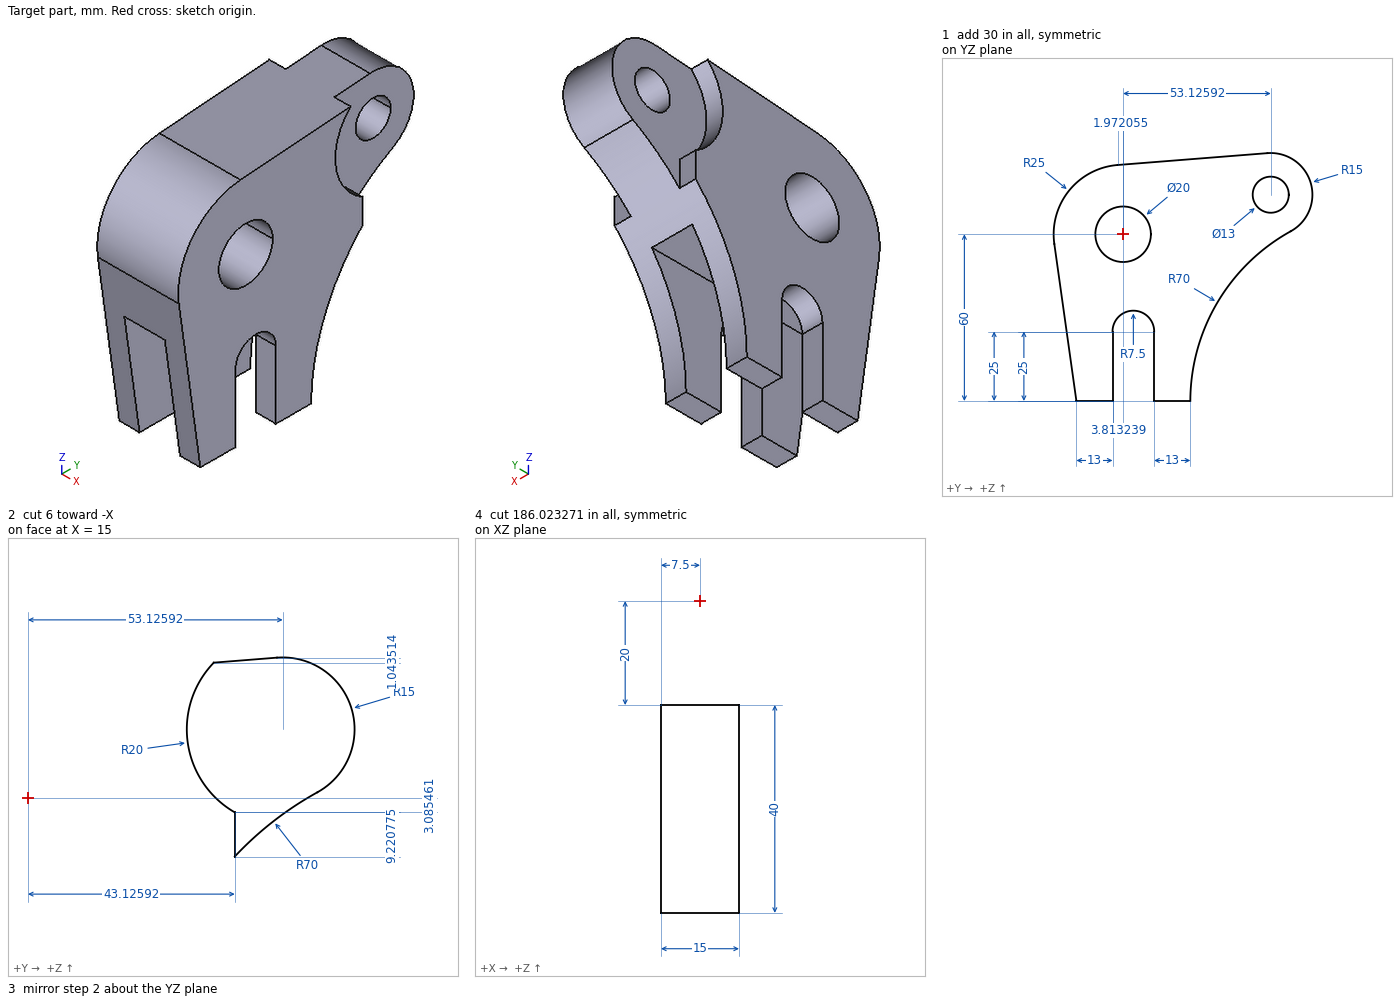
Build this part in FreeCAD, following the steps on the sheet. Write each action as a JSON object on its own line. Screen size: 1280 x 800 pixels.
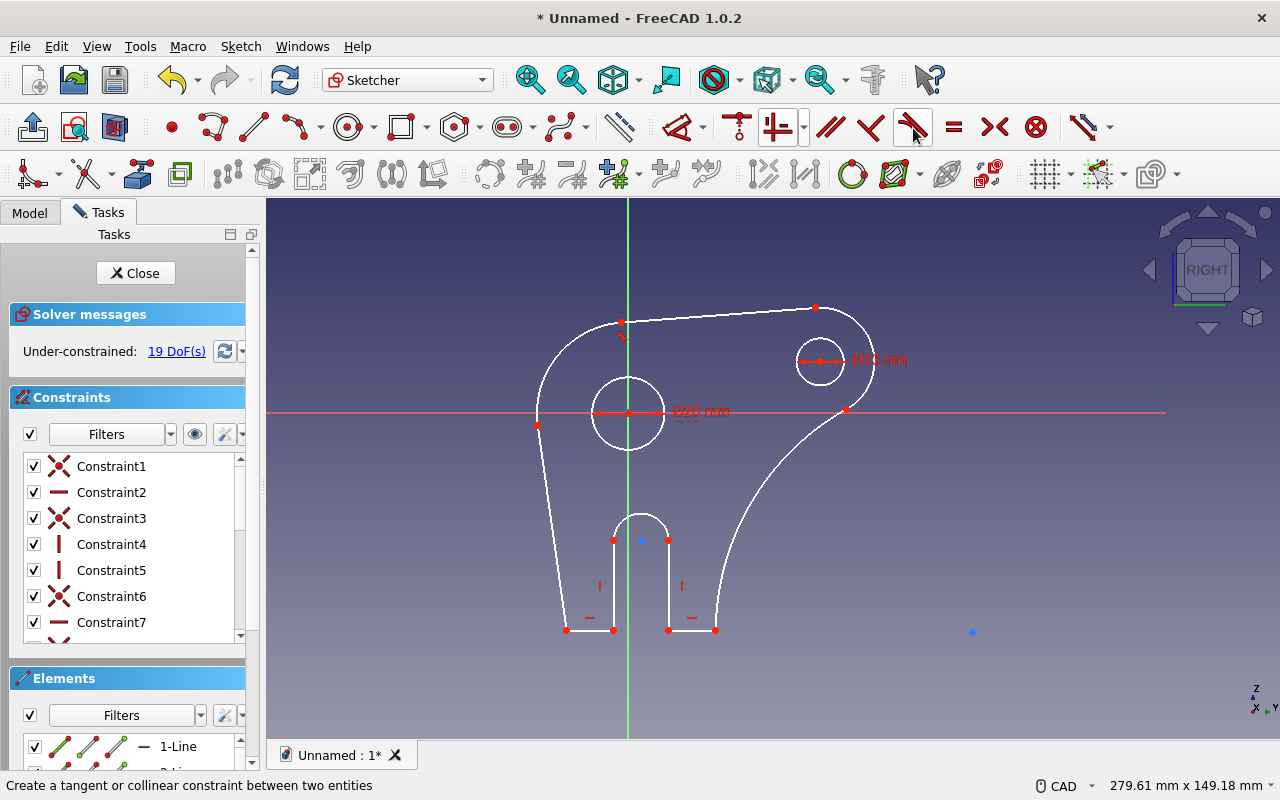
{"action": "left_click", "coordinate": [757, 312]}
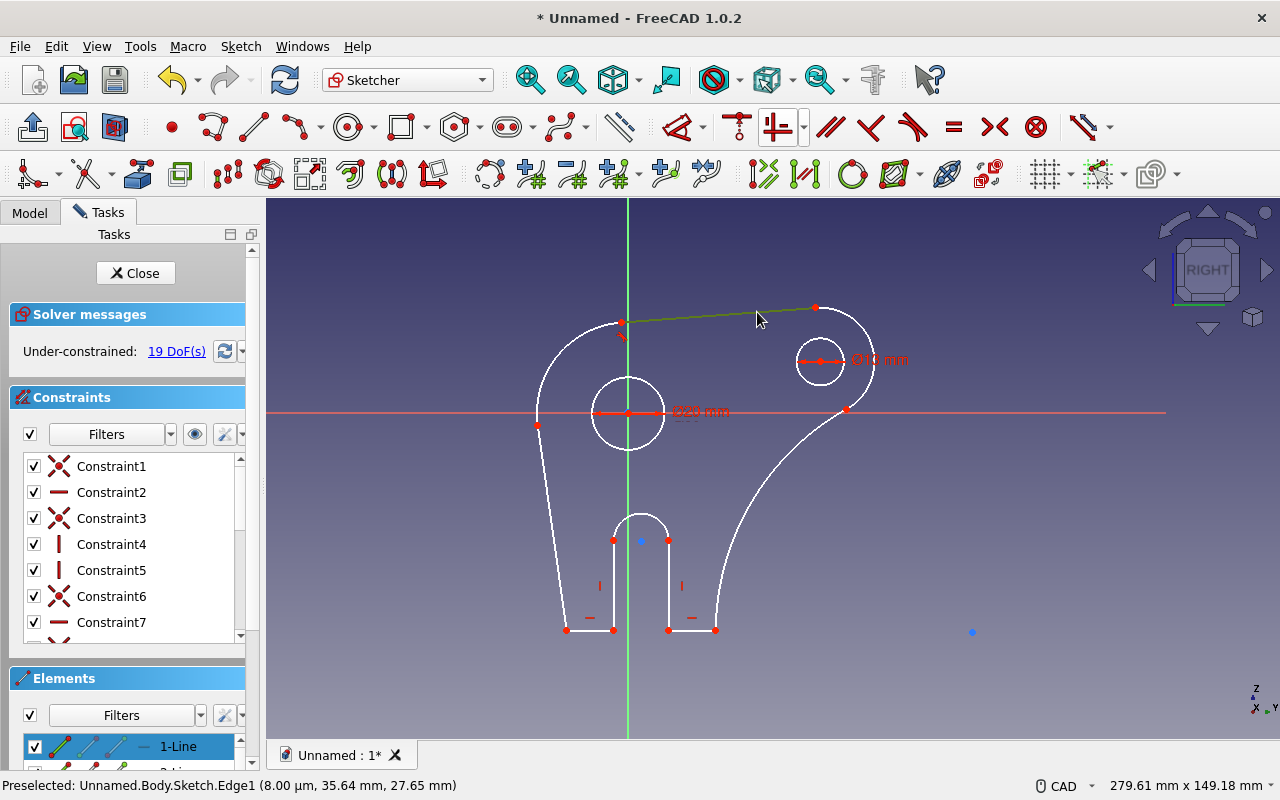
{"action": "left_click", "coordinate": [873, 375]}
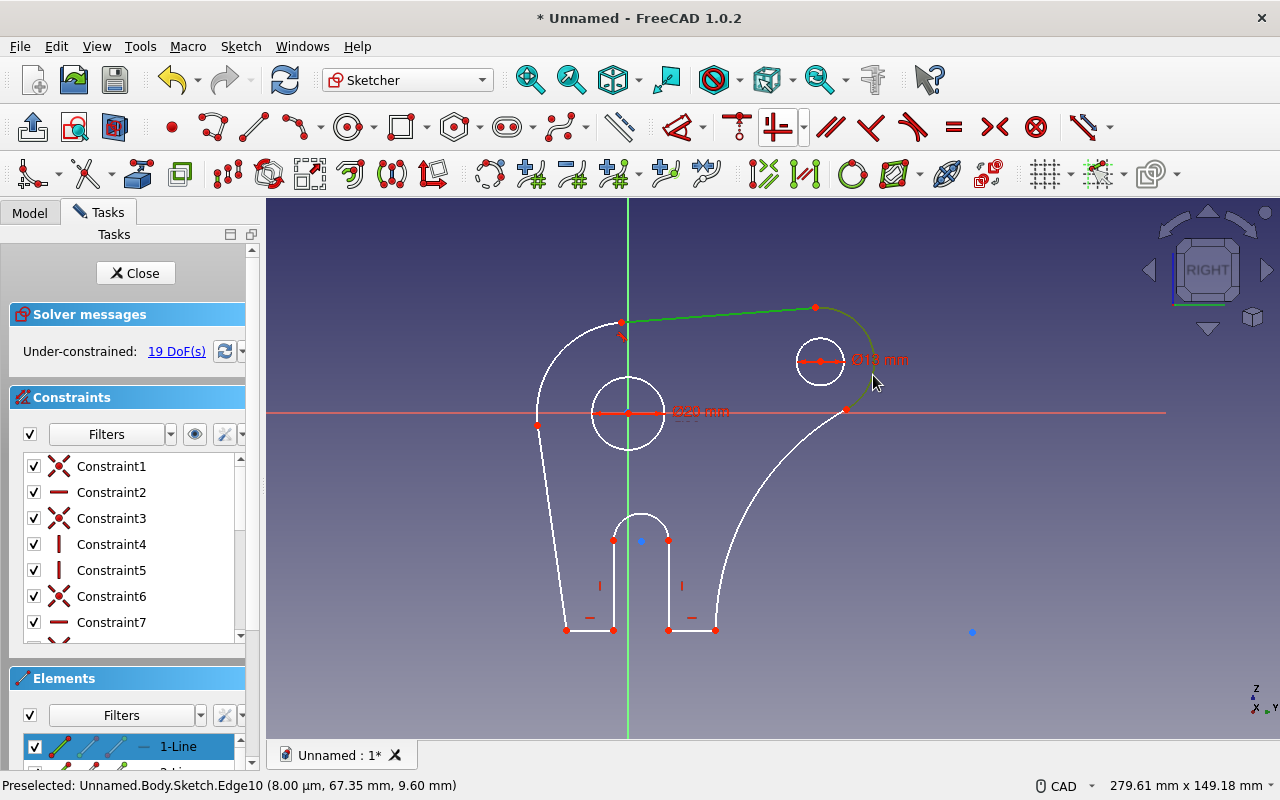
{"action": "left_click", "coordinate": [913, 128]}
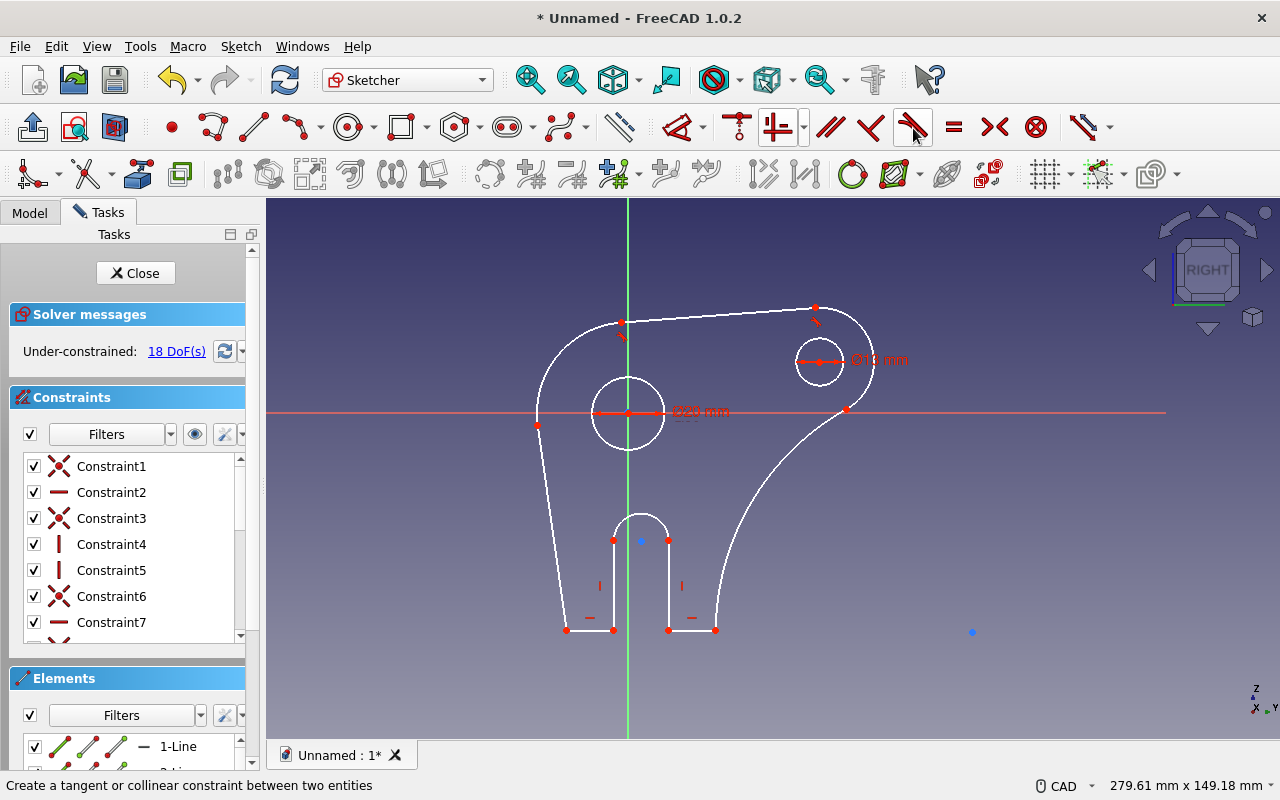
{"action": "left_click", "coordinate": [547, 487]}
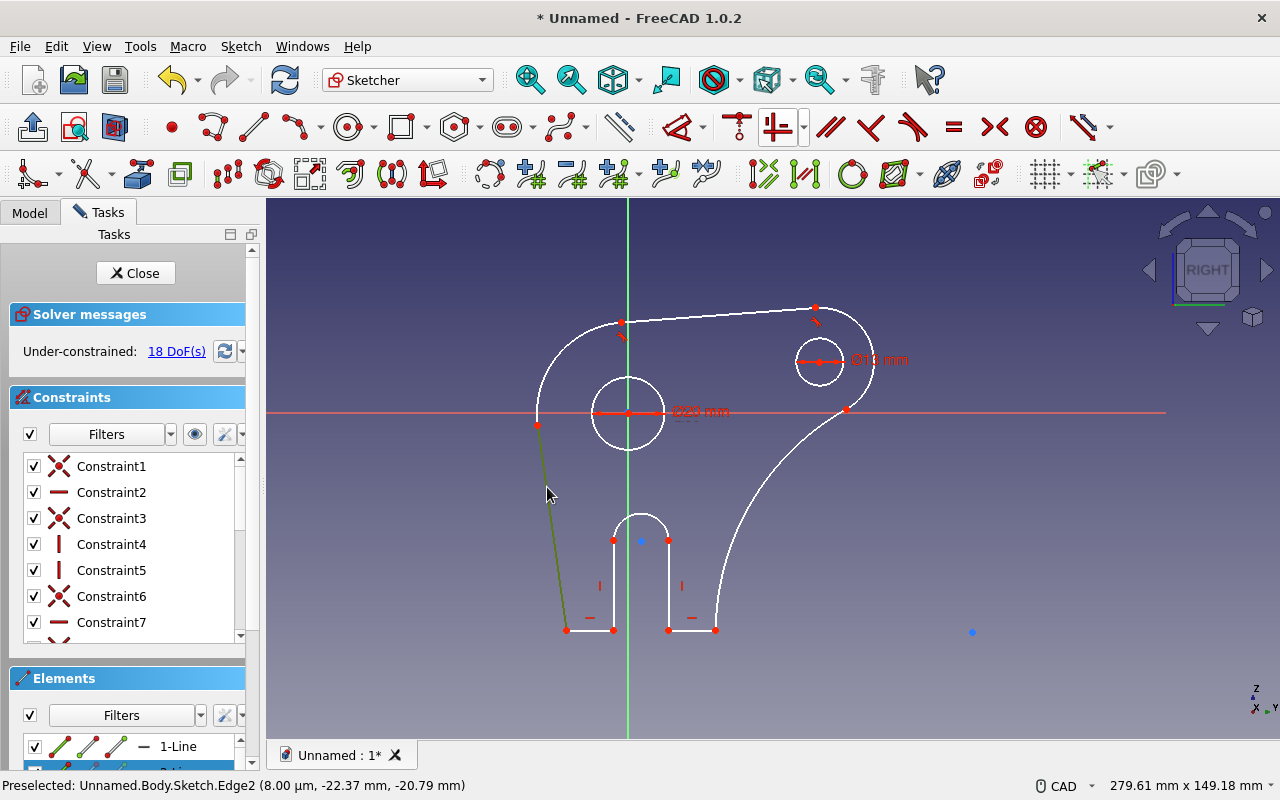
{"action": "left_click", "coordinate": [579, 336]}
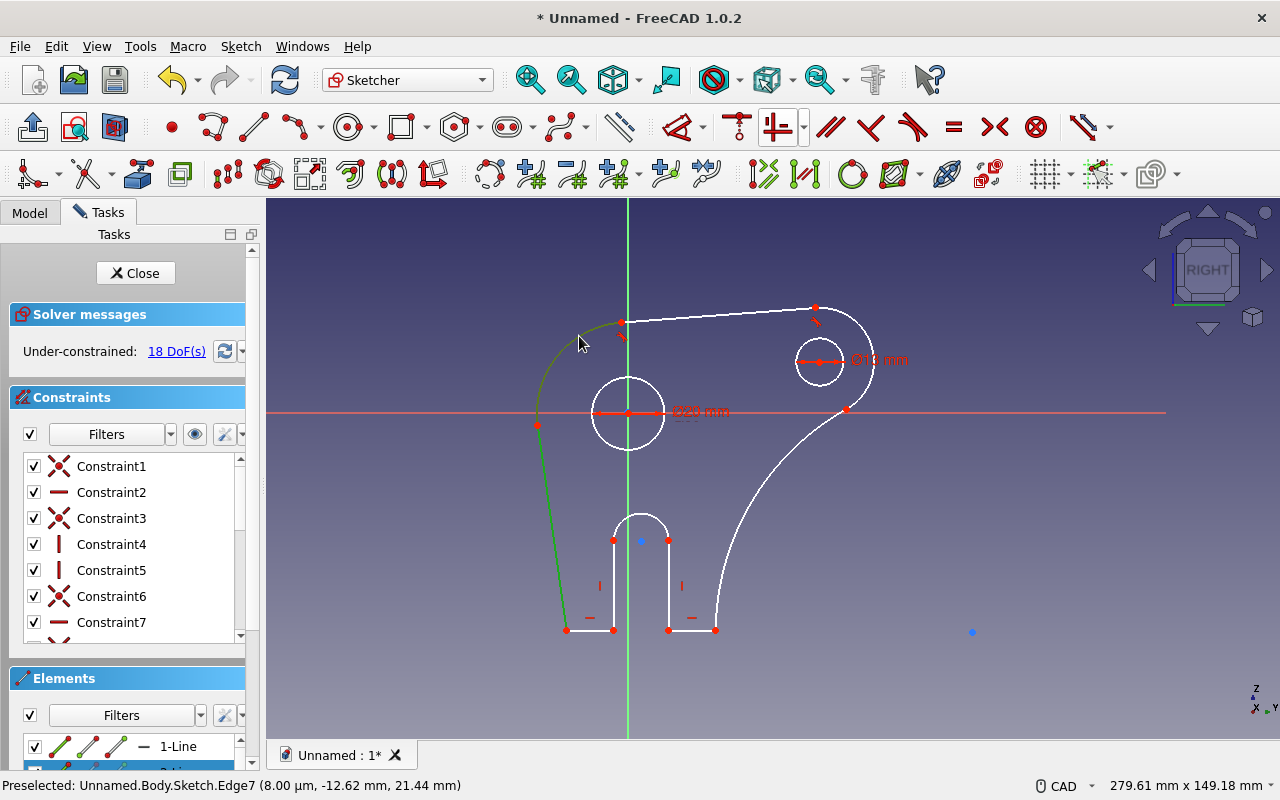
{"action": "left_click", "coordinate": [913, 128]}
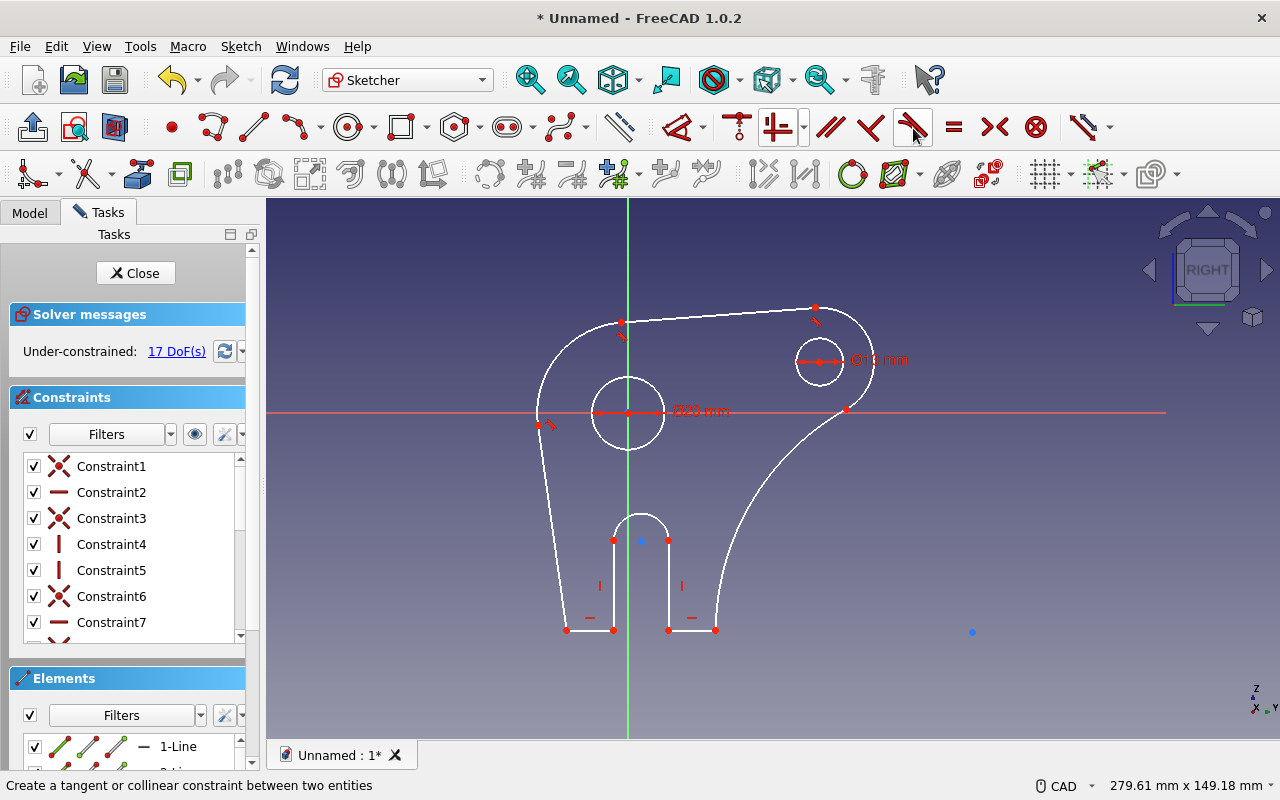
{"action": "left_click", "coordinate": [614, 604]}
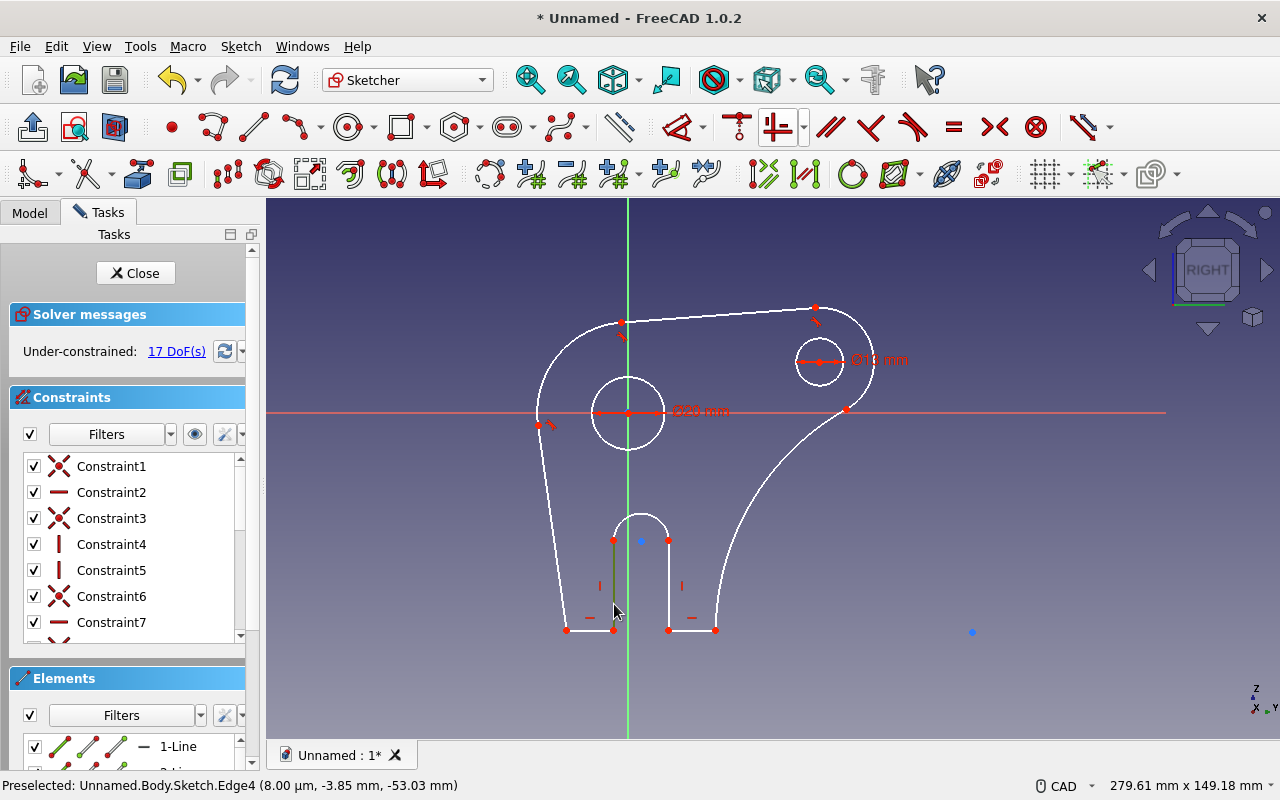
{"action": "left_click", "coordinate": [657, 519]}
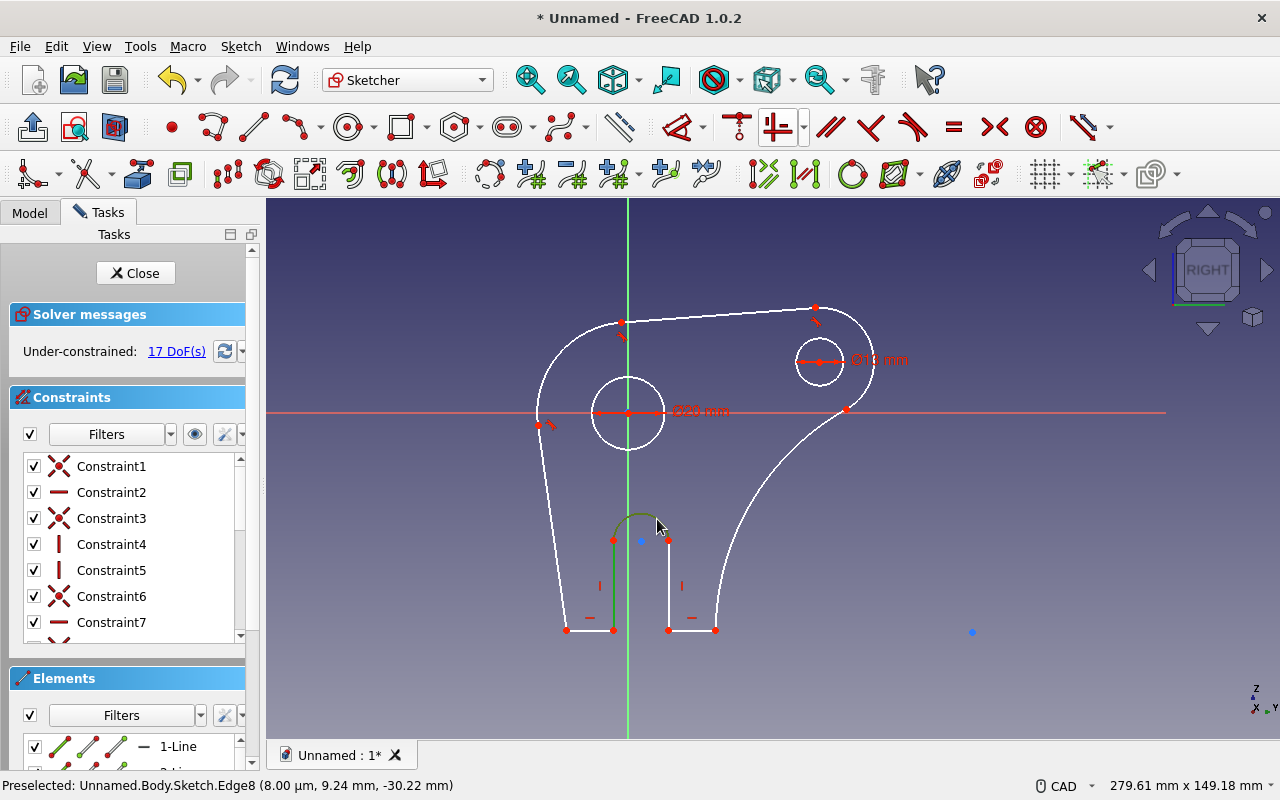
{"action": "left_click", "coordinate": [913, 128]}